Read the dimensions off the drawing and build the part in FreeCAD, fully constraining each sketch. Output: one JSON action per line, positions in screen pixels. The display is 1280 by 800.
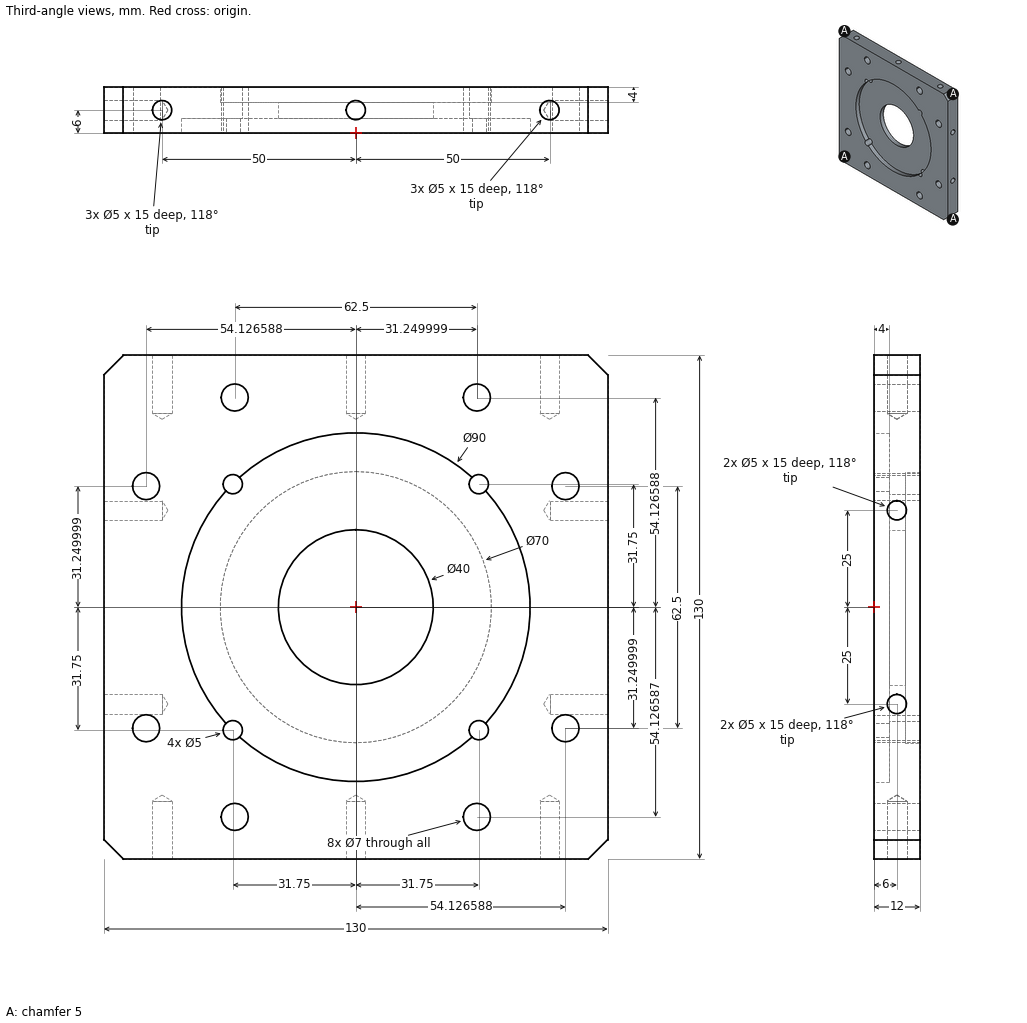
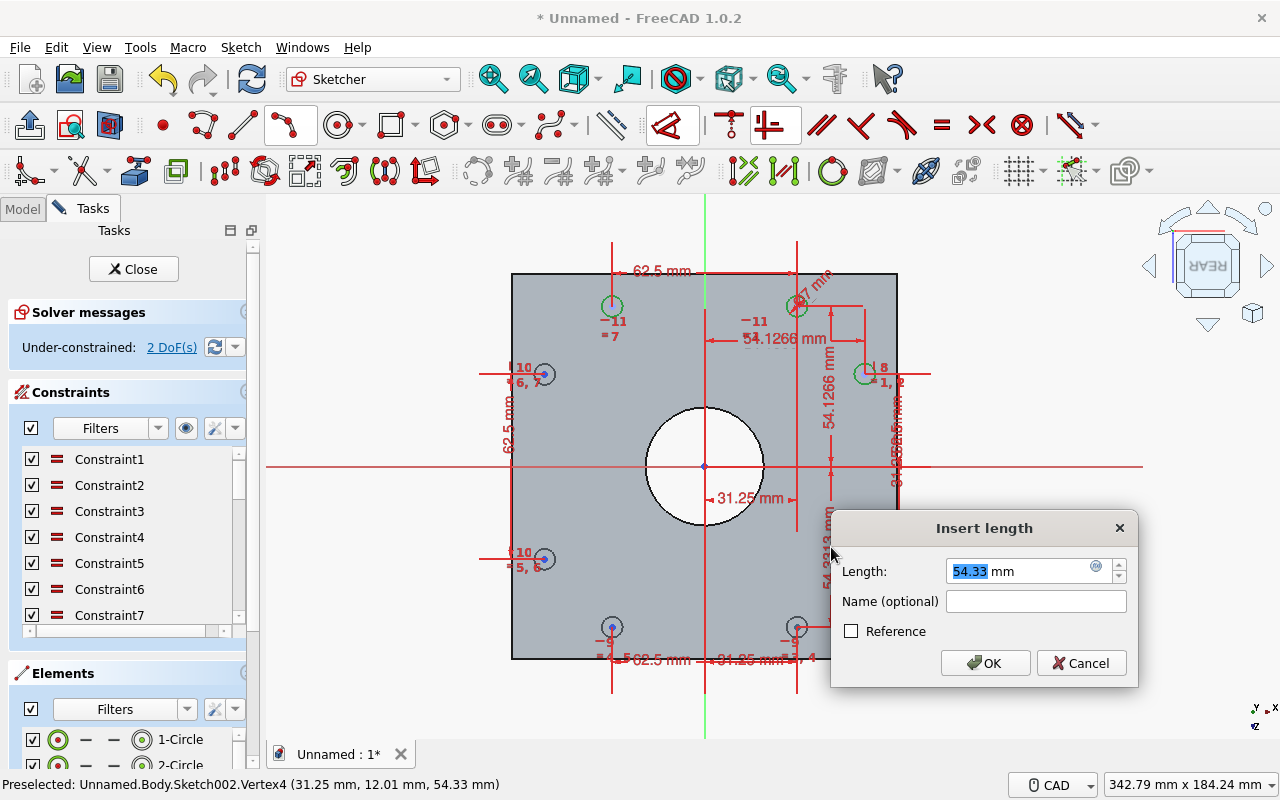
{"action": "type", "text": "54.126588"}
{"action": "key", "text": "Return"}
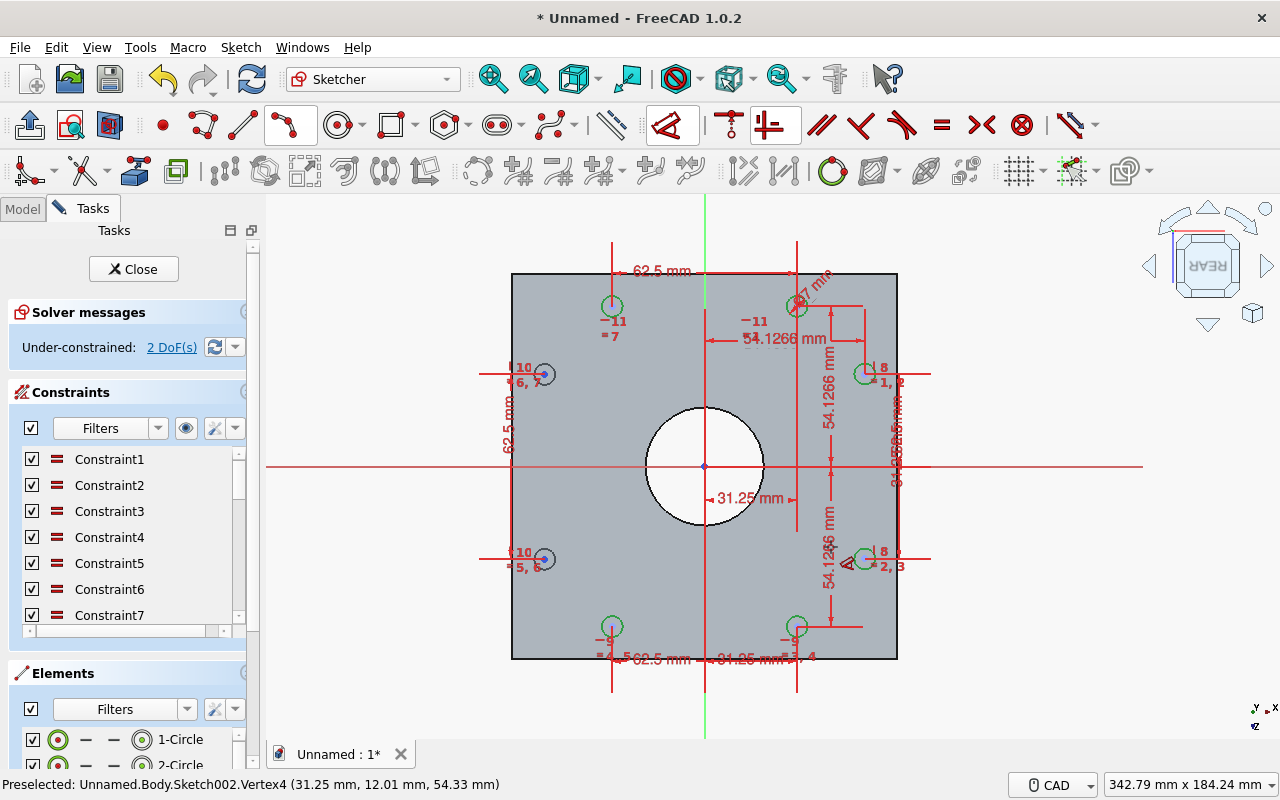
{"action": "left_click", "coordinate": [545, 559]}
{"action": "left_click", "coordinate": [625, 593]}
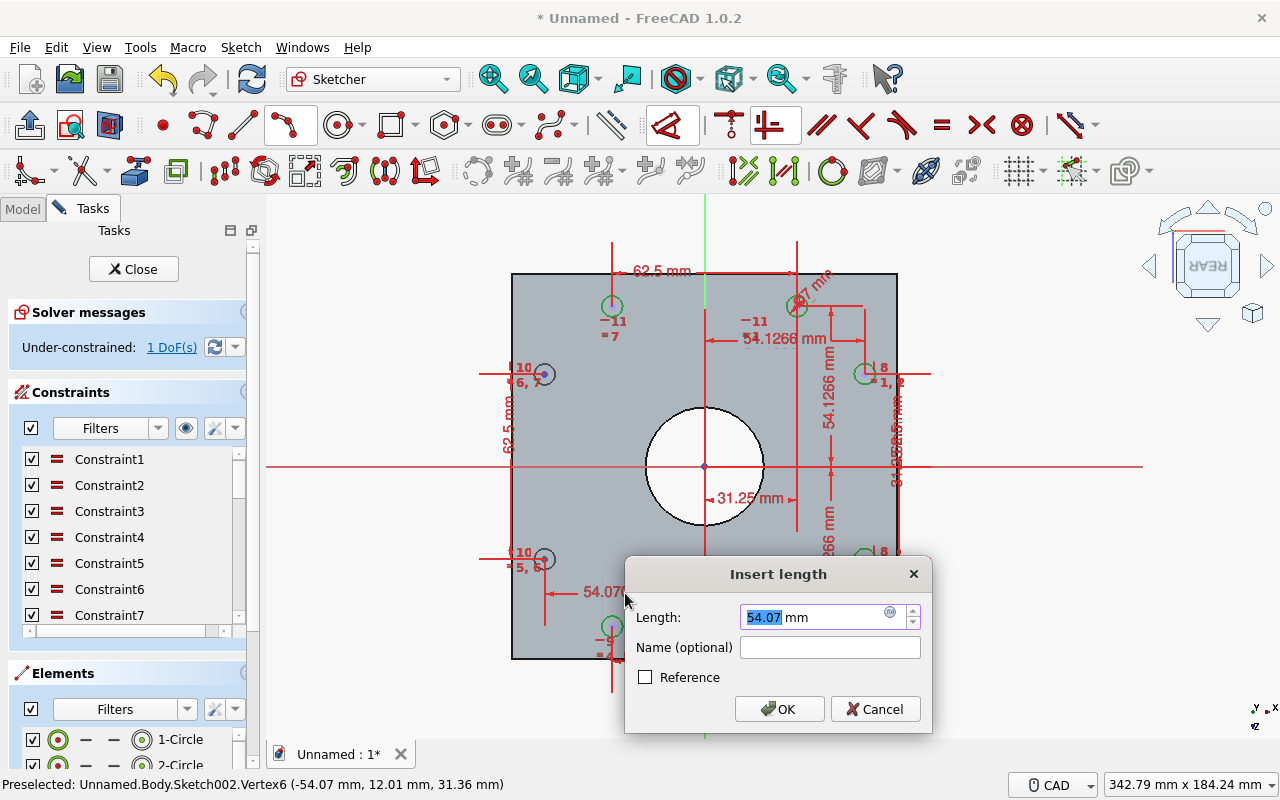
{"action": "type", "text": "54.126588"}
{"action": "key", "text": "Return"}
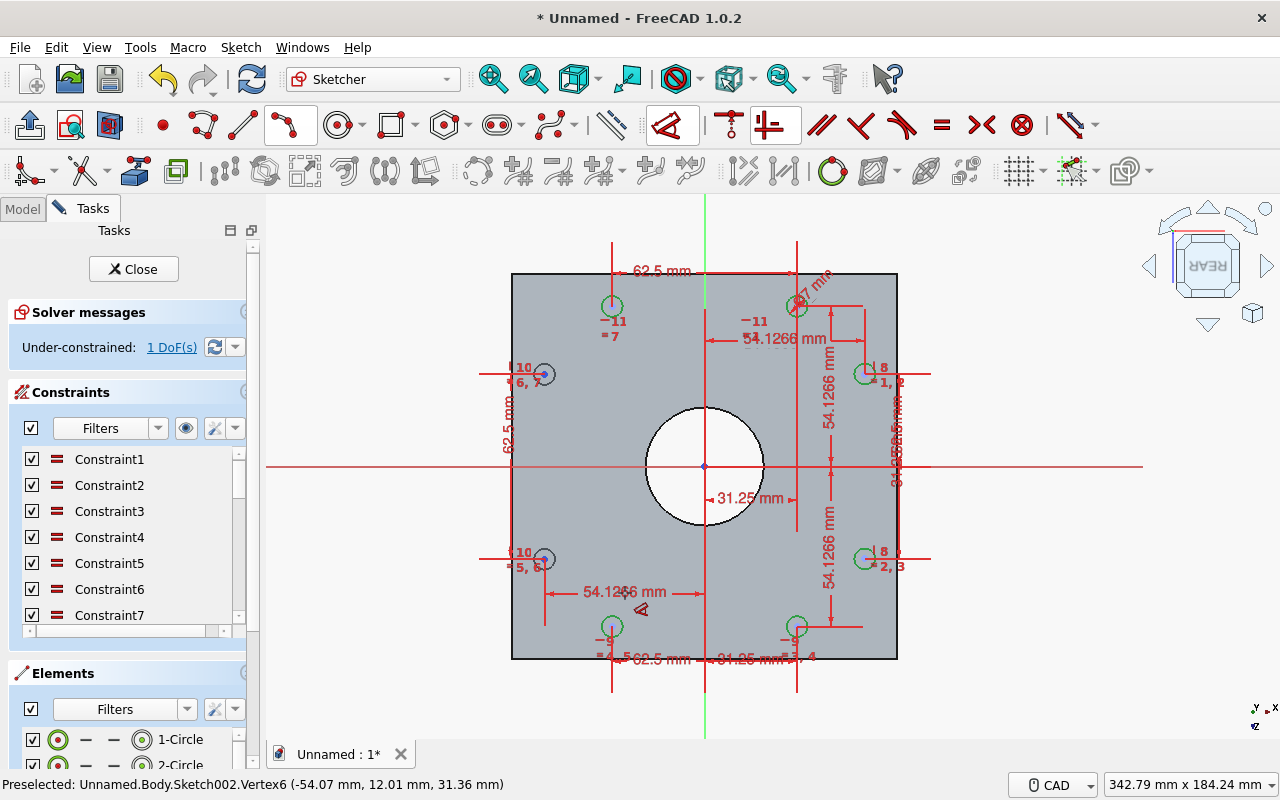
{"action": "left_click", "coordinate": [545, 559]}
{"action": "left_click", "coordinate": [511, 513]}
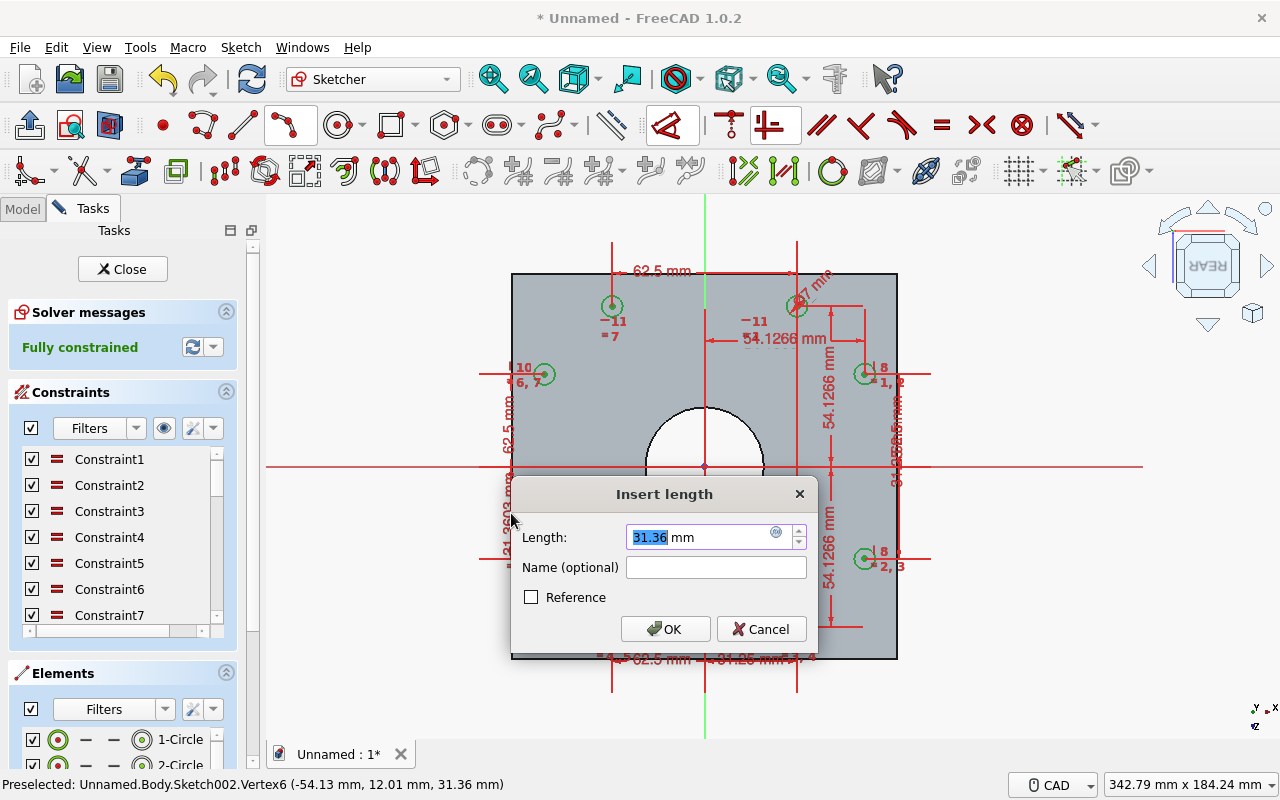
{"action": "type", "text": "31.249999"}
{"action": "key", "text": "Return"}
{"action": "key", "text": "Escape"}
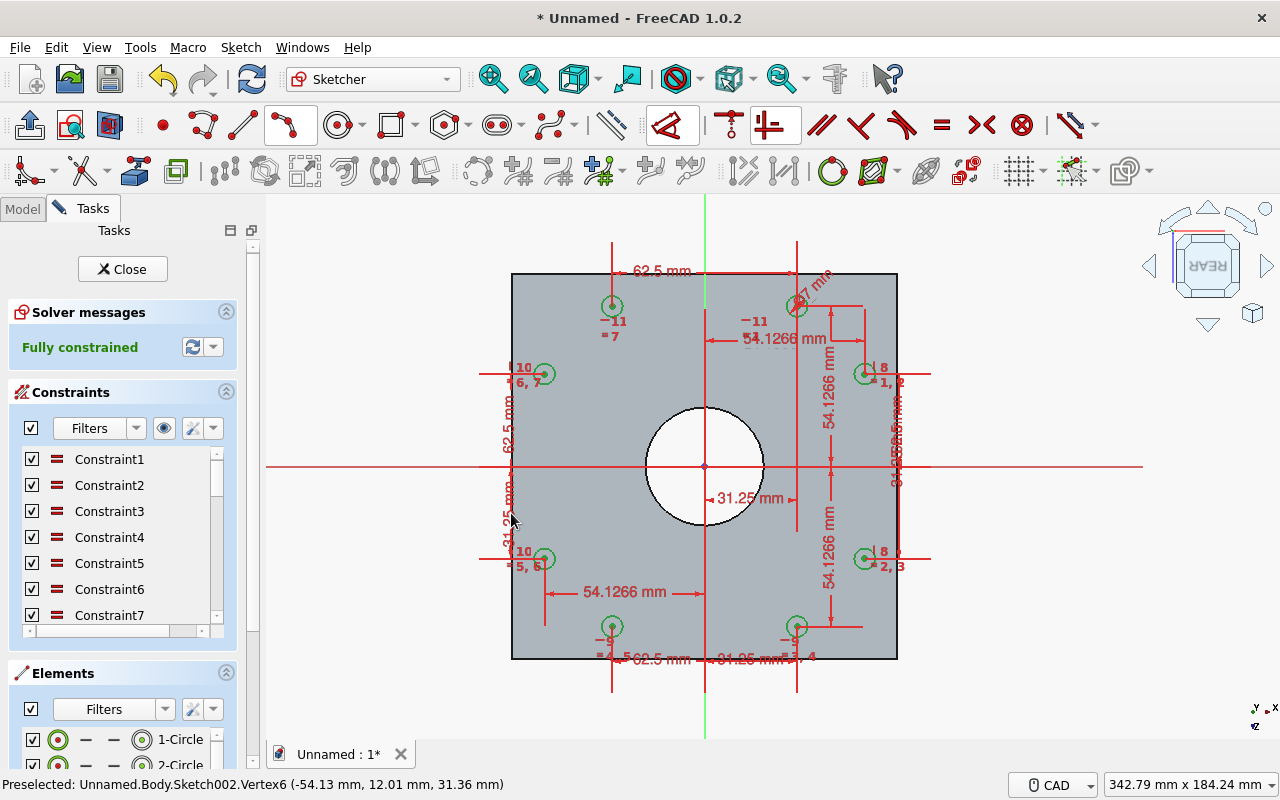
{"action": "left_click", "coordinate": [123, 269]}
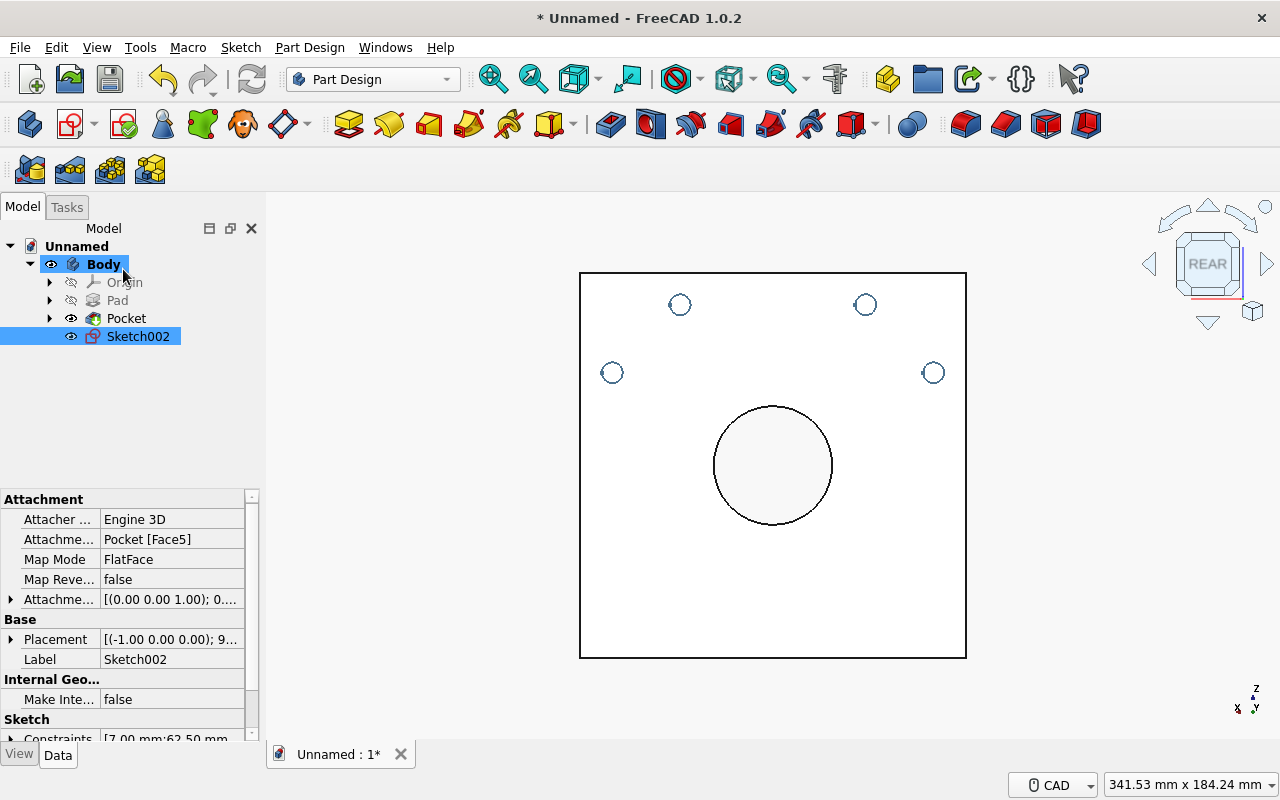
{"action": "left_click", "coordinate": [652, 124]}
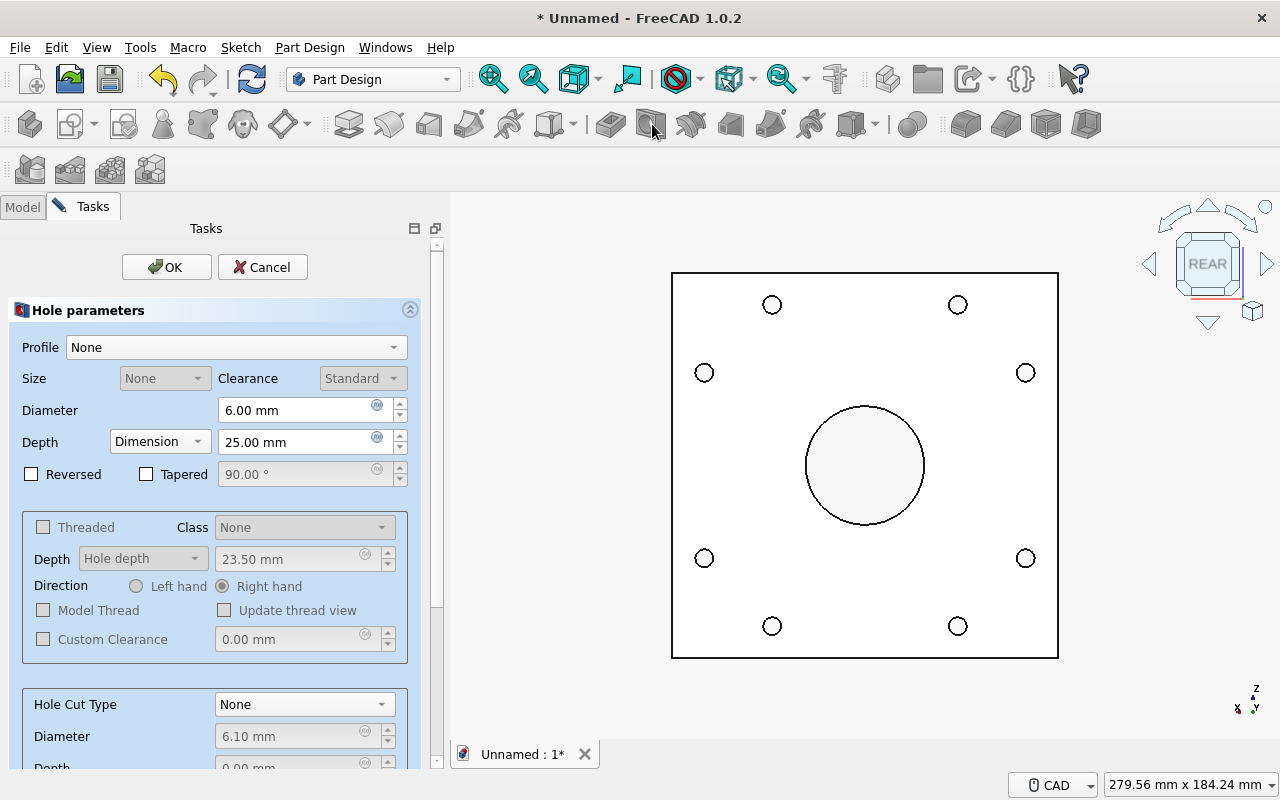
{"action": "triple_click", "coordinate": [305, 410]}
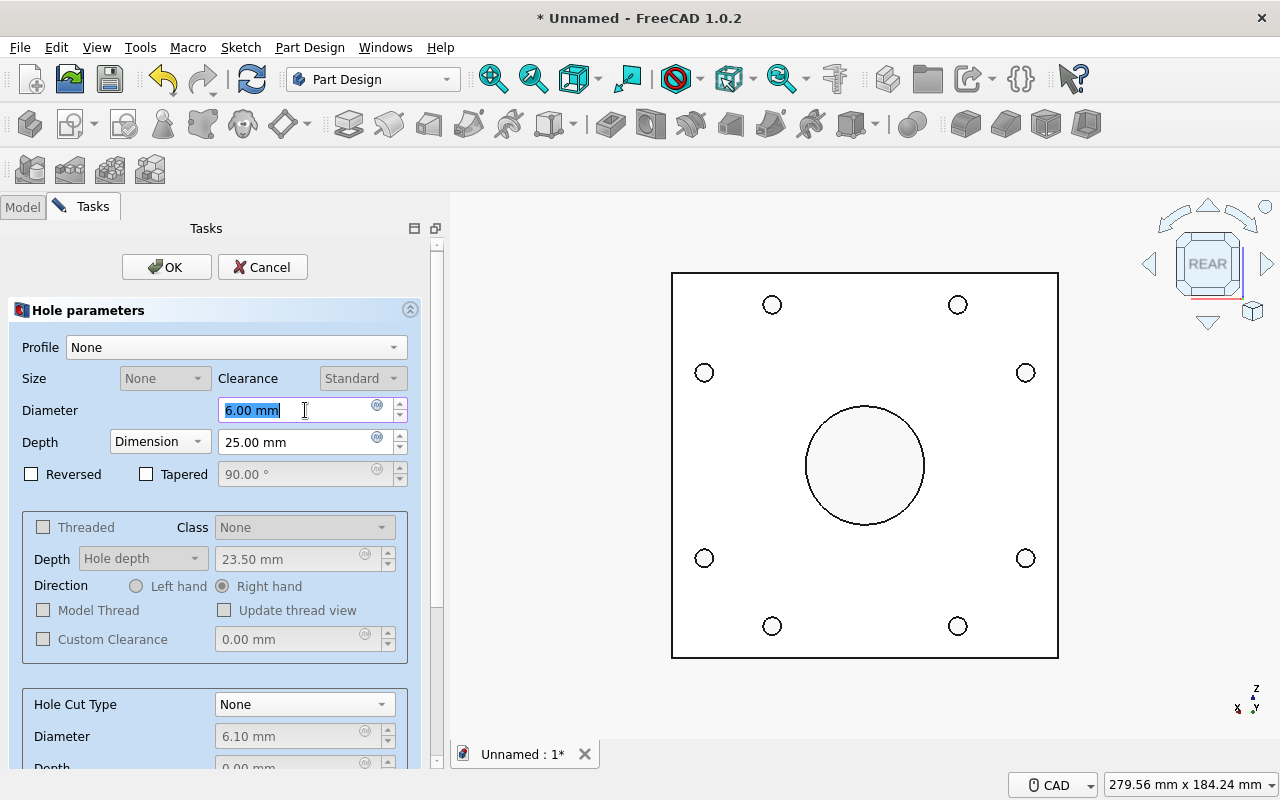
{"action": "type", "text": "7"}
{"action": "key", "text": "Tab"}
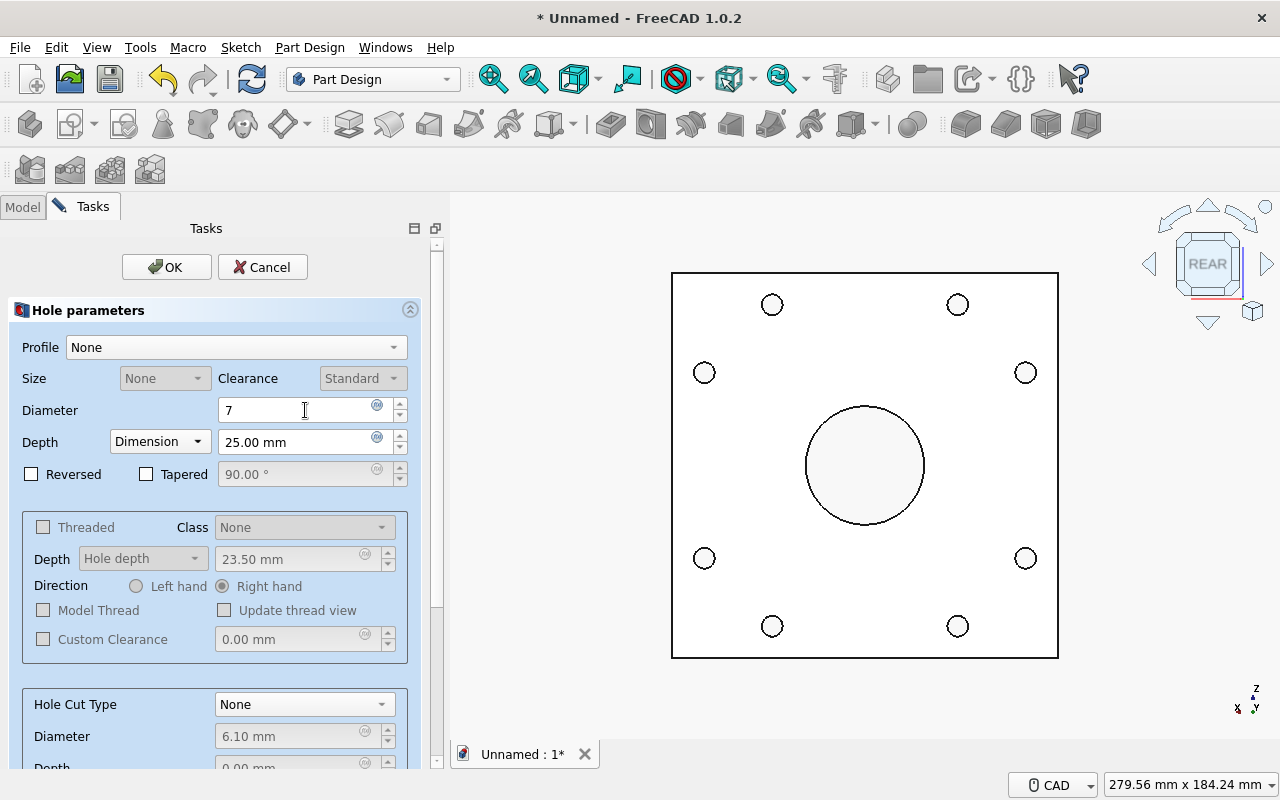
{"action": "left_click", "coordinate": [161, 442]}